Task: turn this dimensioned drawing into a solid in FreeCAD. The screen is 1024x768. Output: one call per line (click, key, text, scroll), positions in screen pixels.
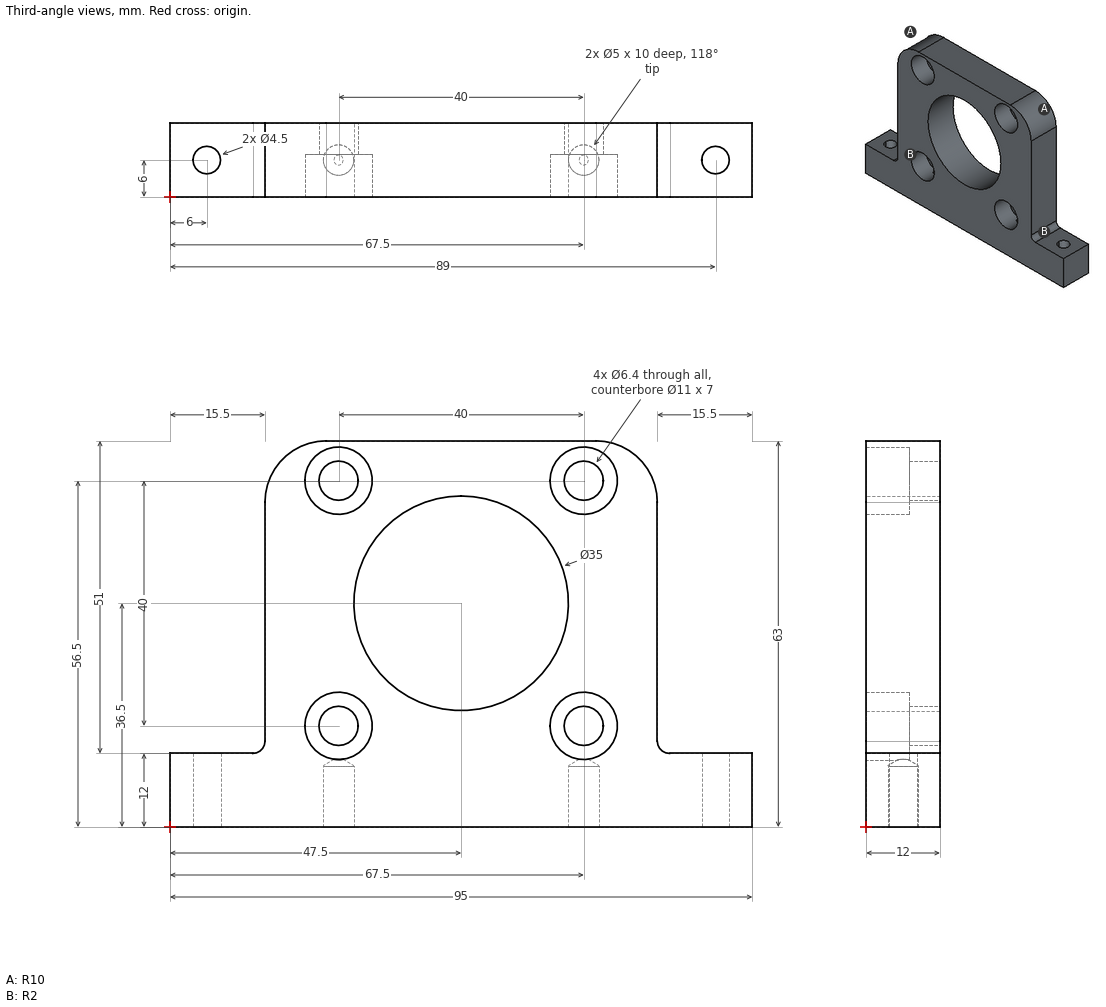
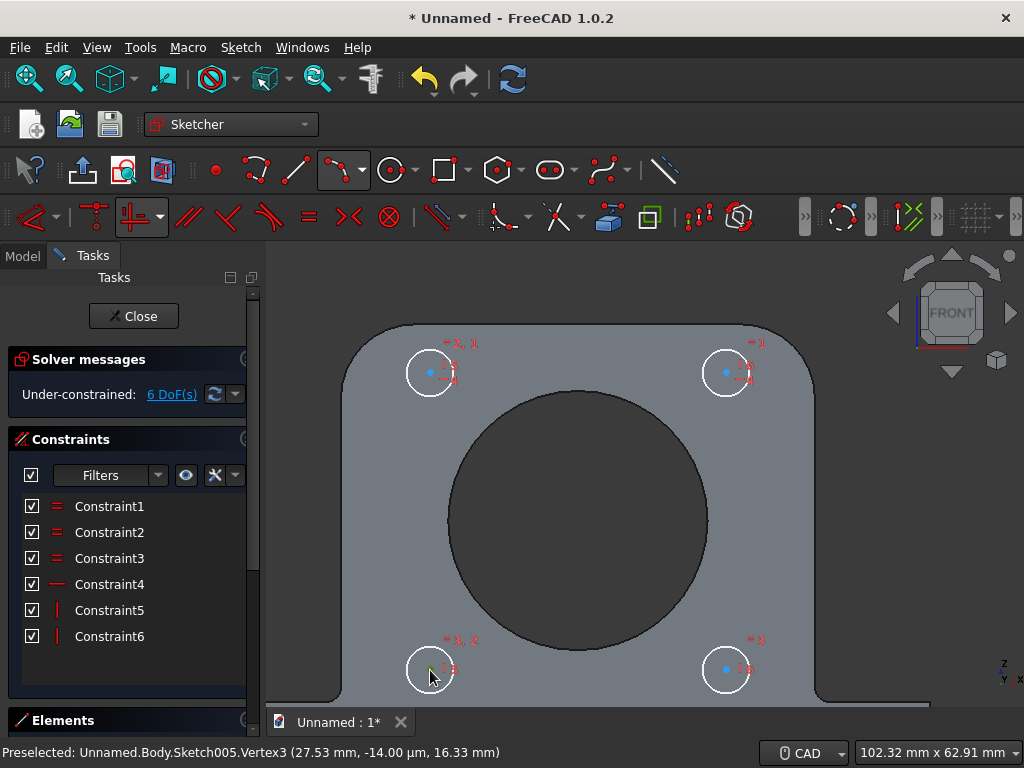
click(726, 670)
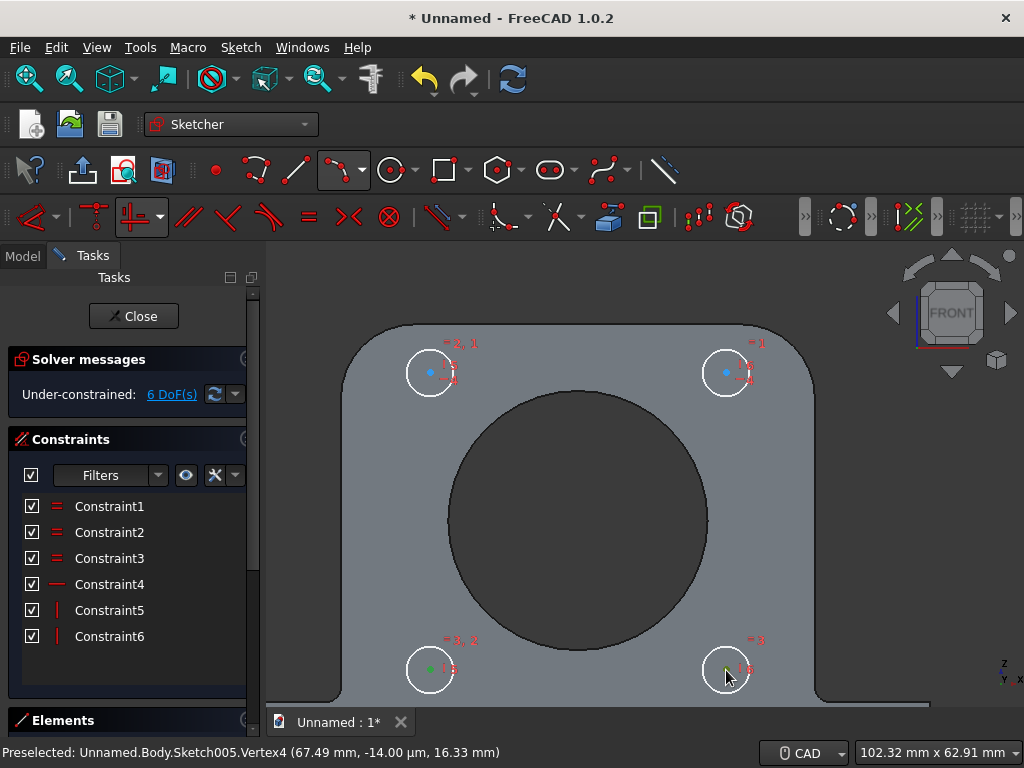
click(162, 218)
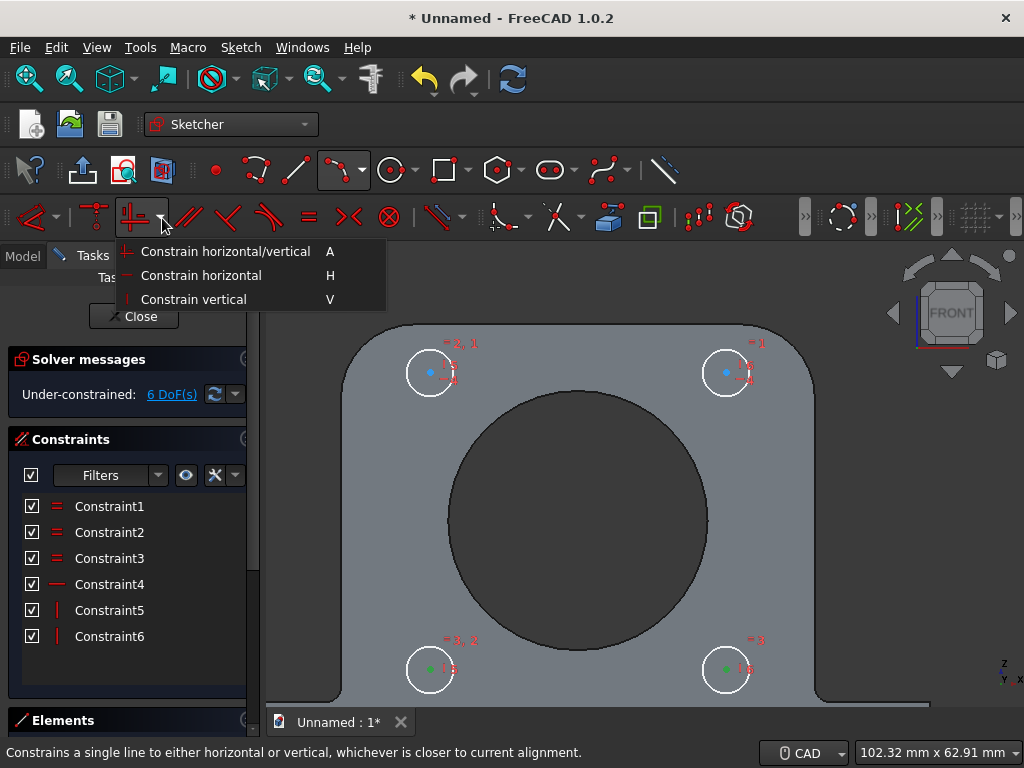
click(251, 275)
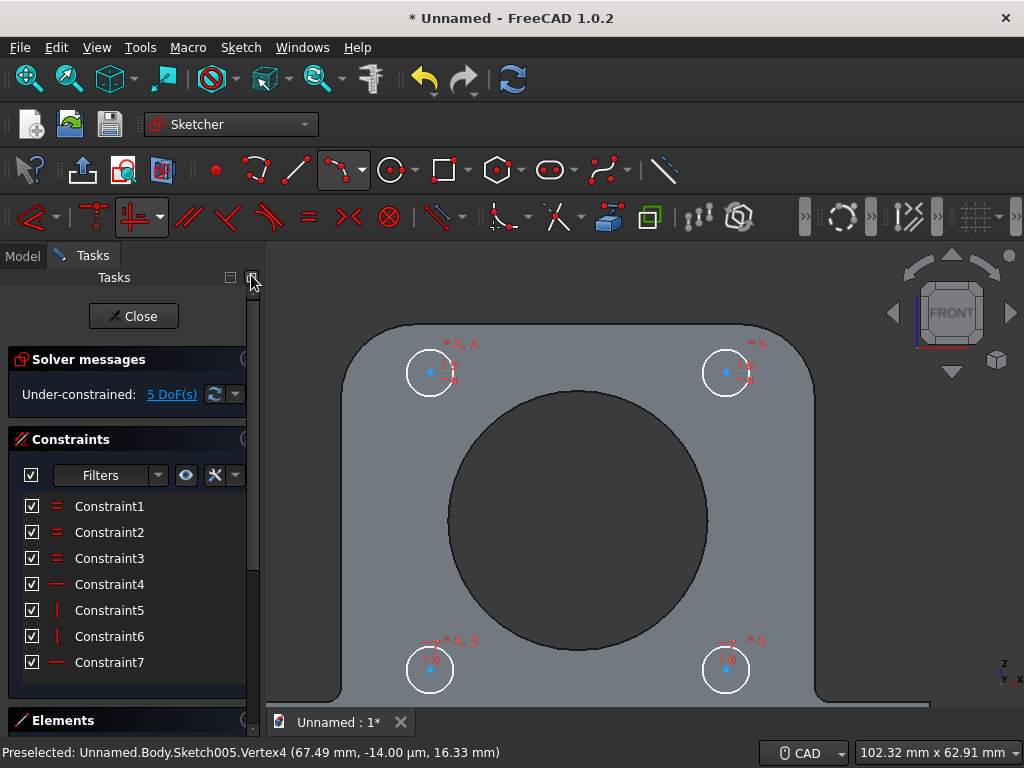
click(32, 218)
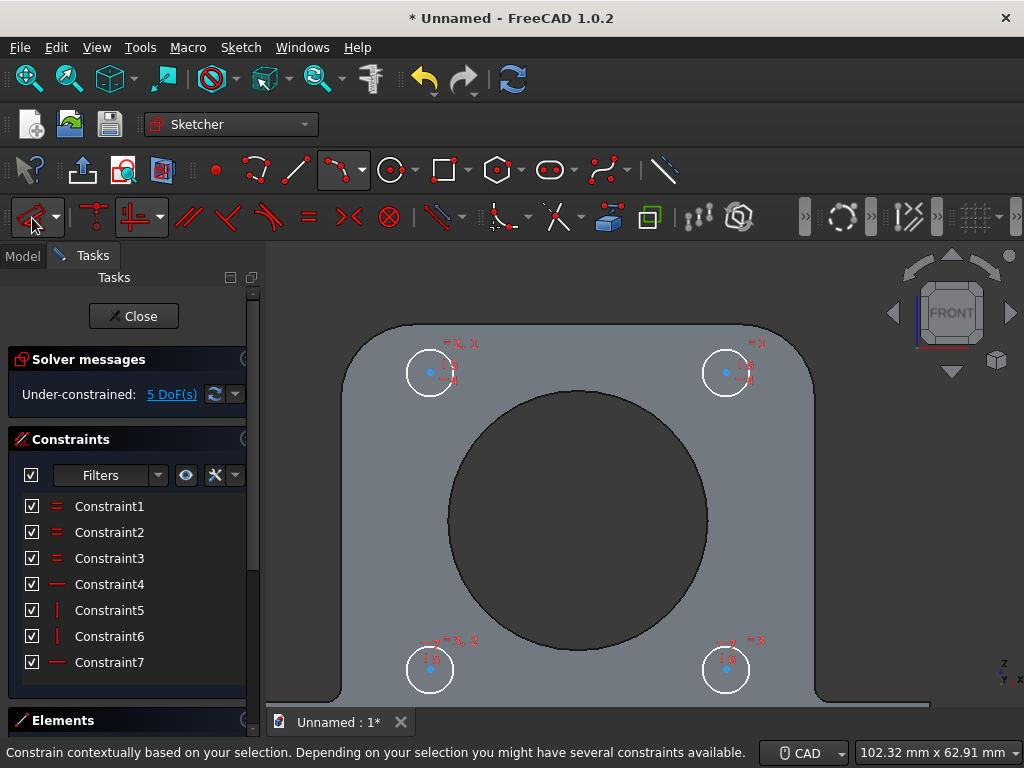
click(742, 356)
click(764, 333)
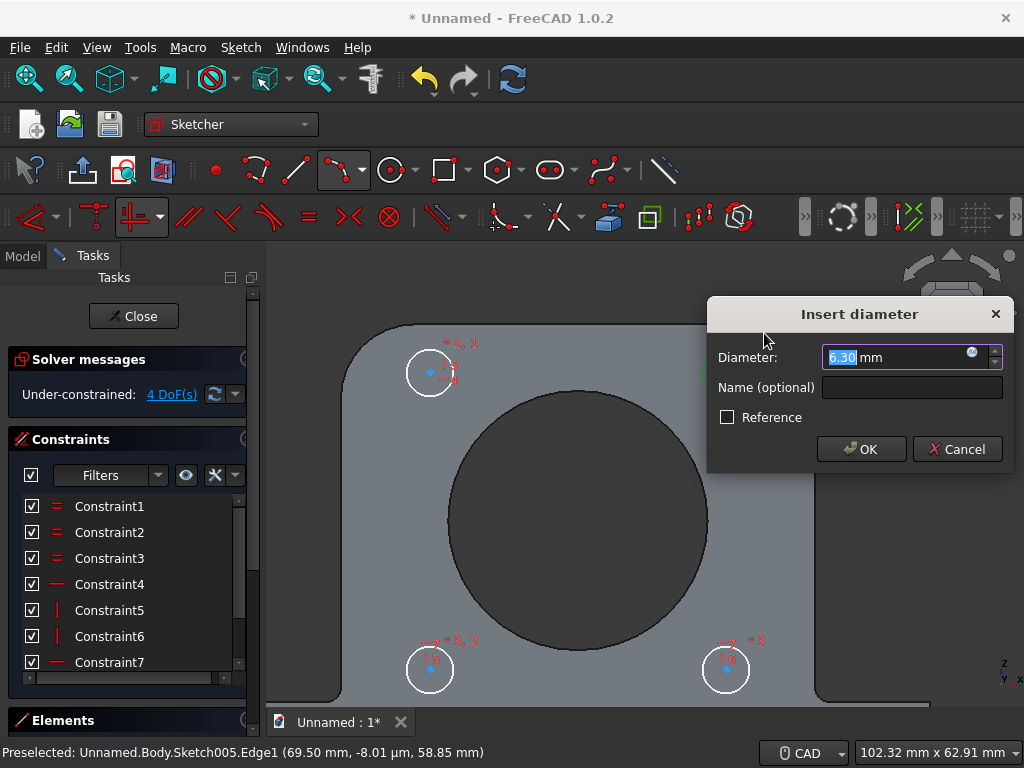
text(6.4)
key(Return)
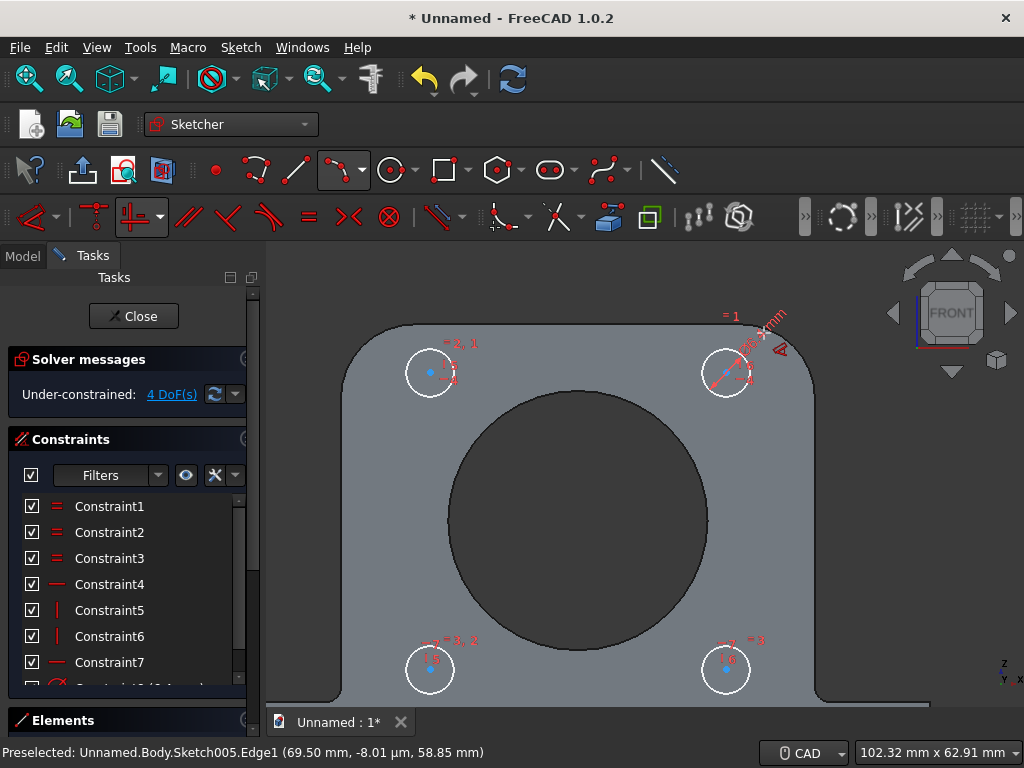
click(726, 373)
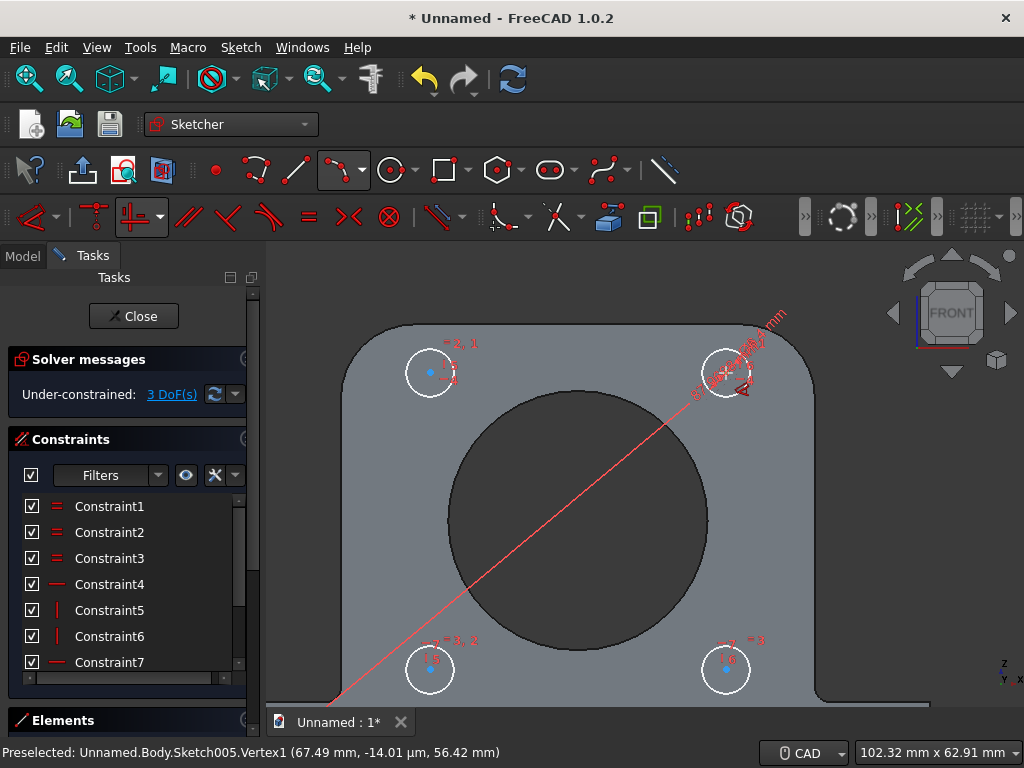
click(430, 373)
click(578, 339)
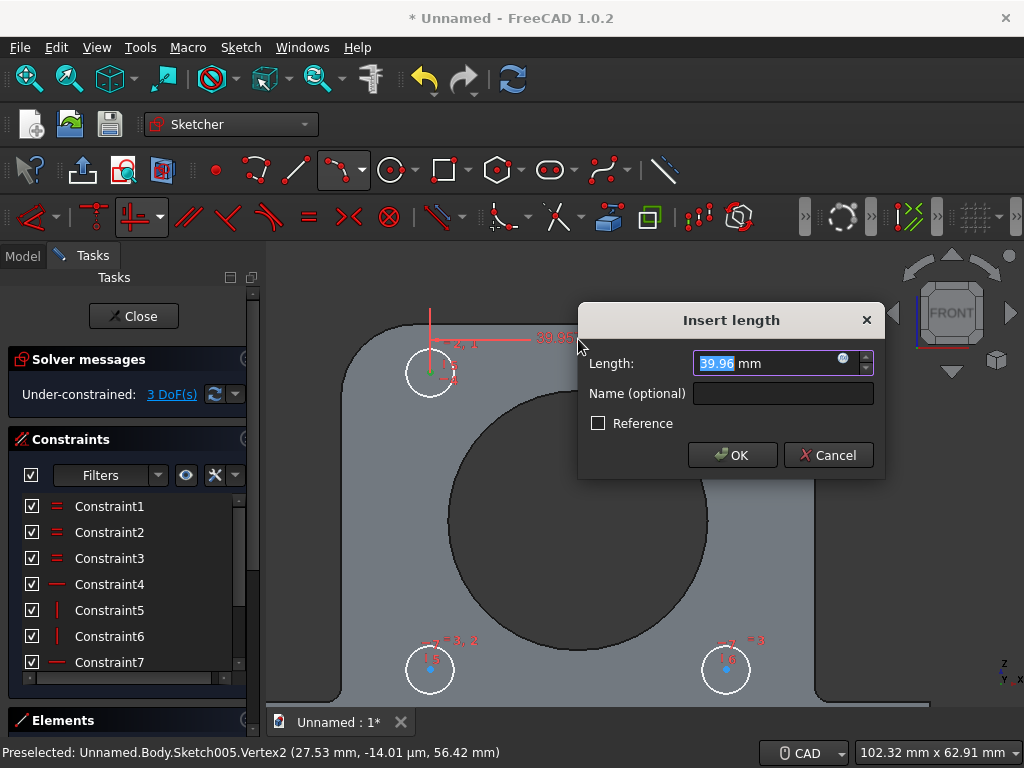
text(40)
key(Return)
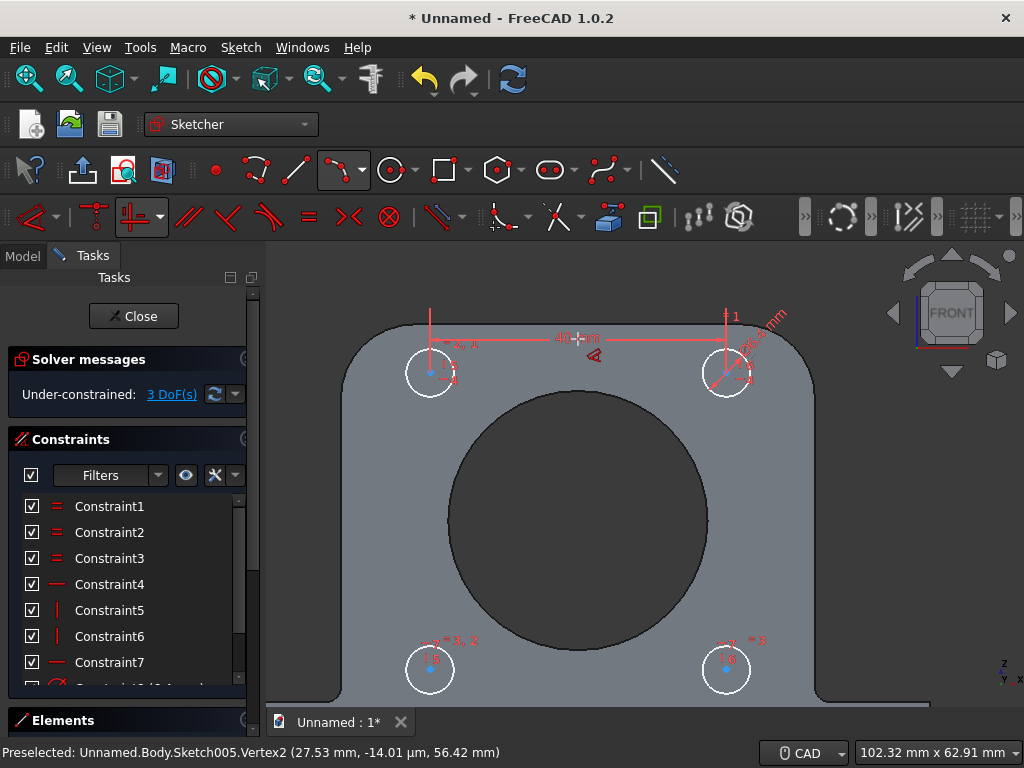
click(430, 373)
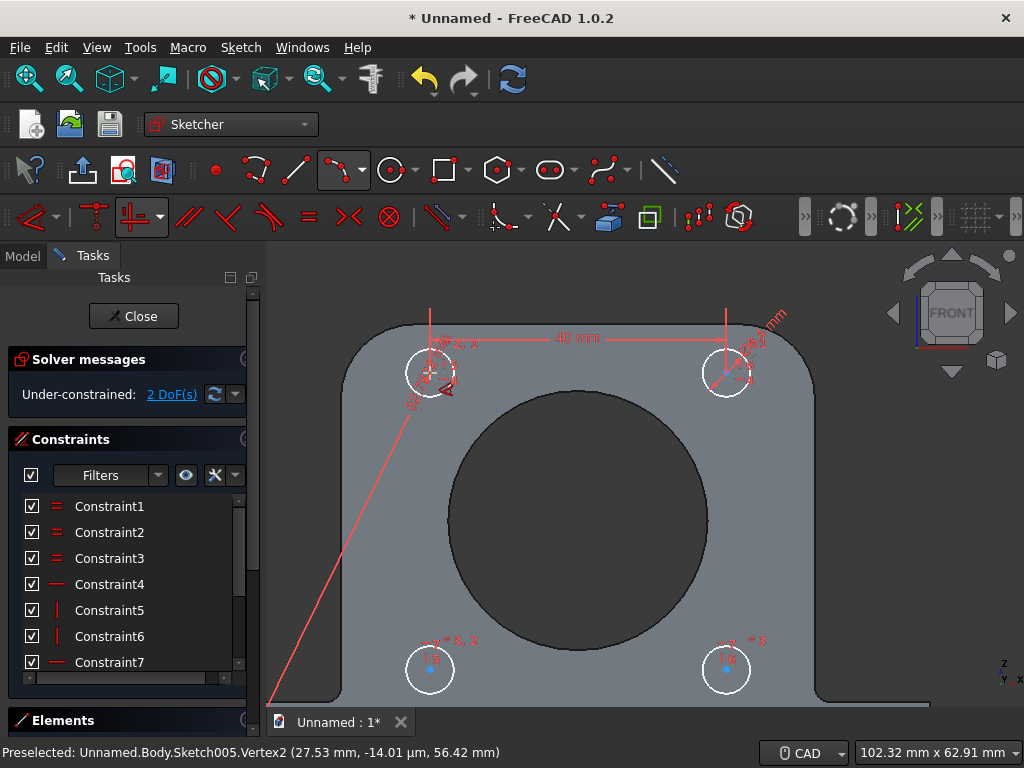
click(430, 670)
click(396, 521)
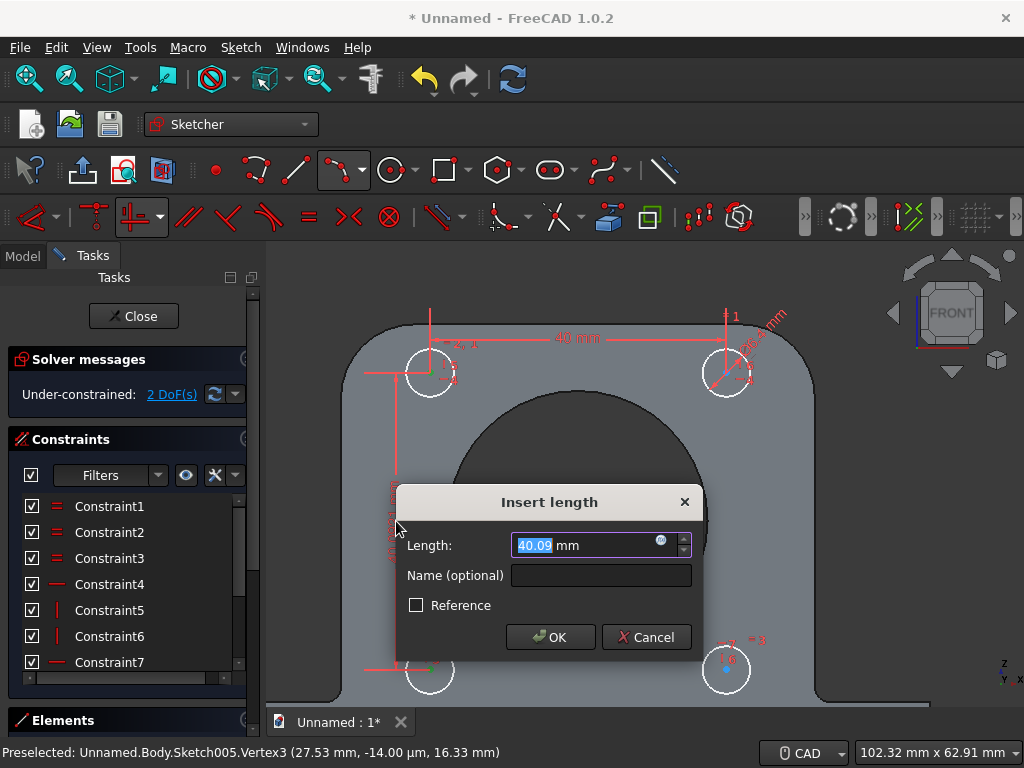
text(40)
key(Return)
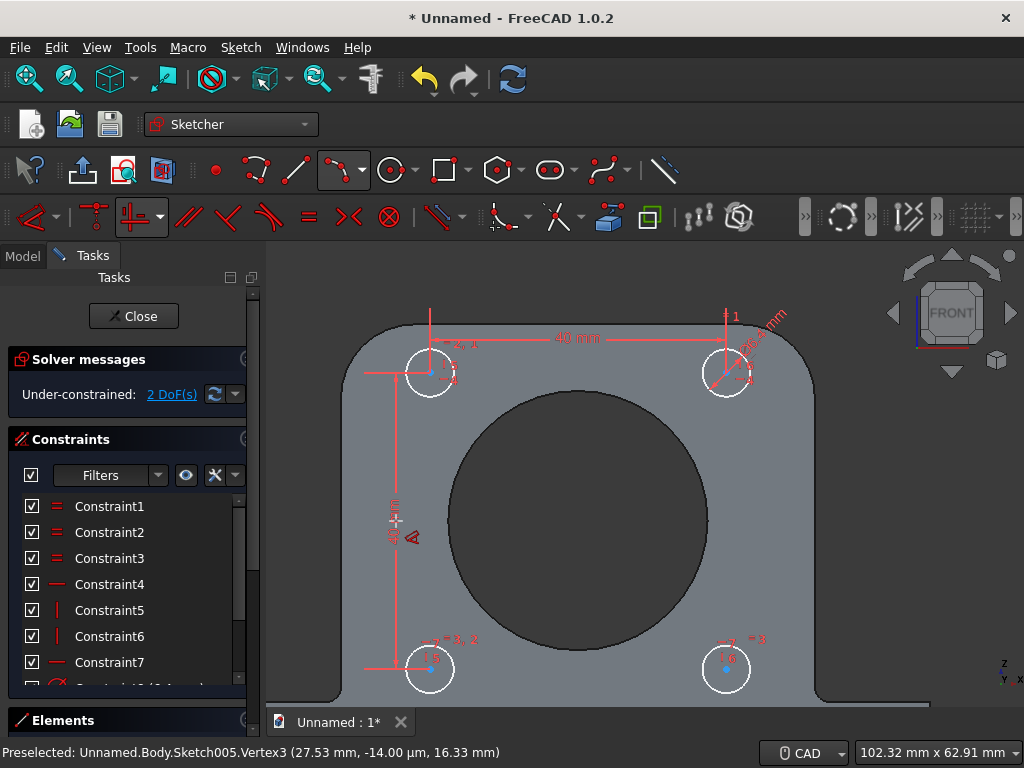
click(726, 373)
click(411, 339)